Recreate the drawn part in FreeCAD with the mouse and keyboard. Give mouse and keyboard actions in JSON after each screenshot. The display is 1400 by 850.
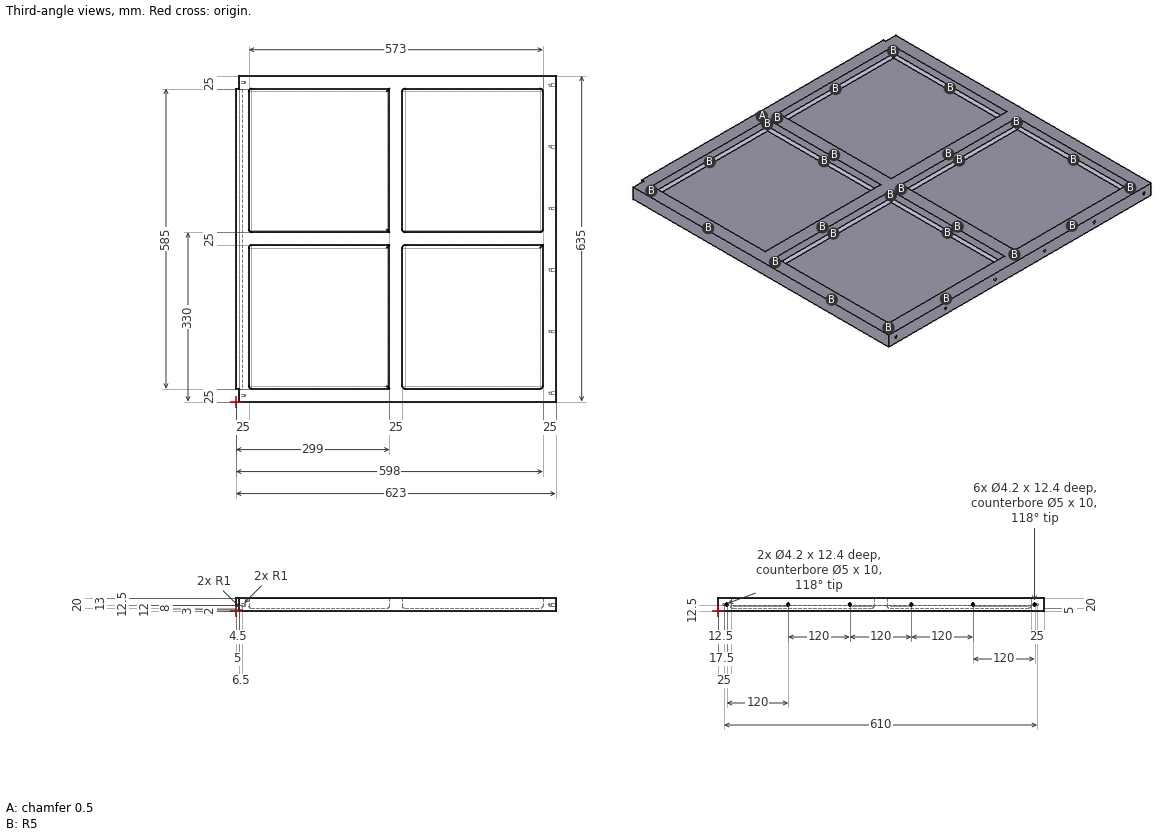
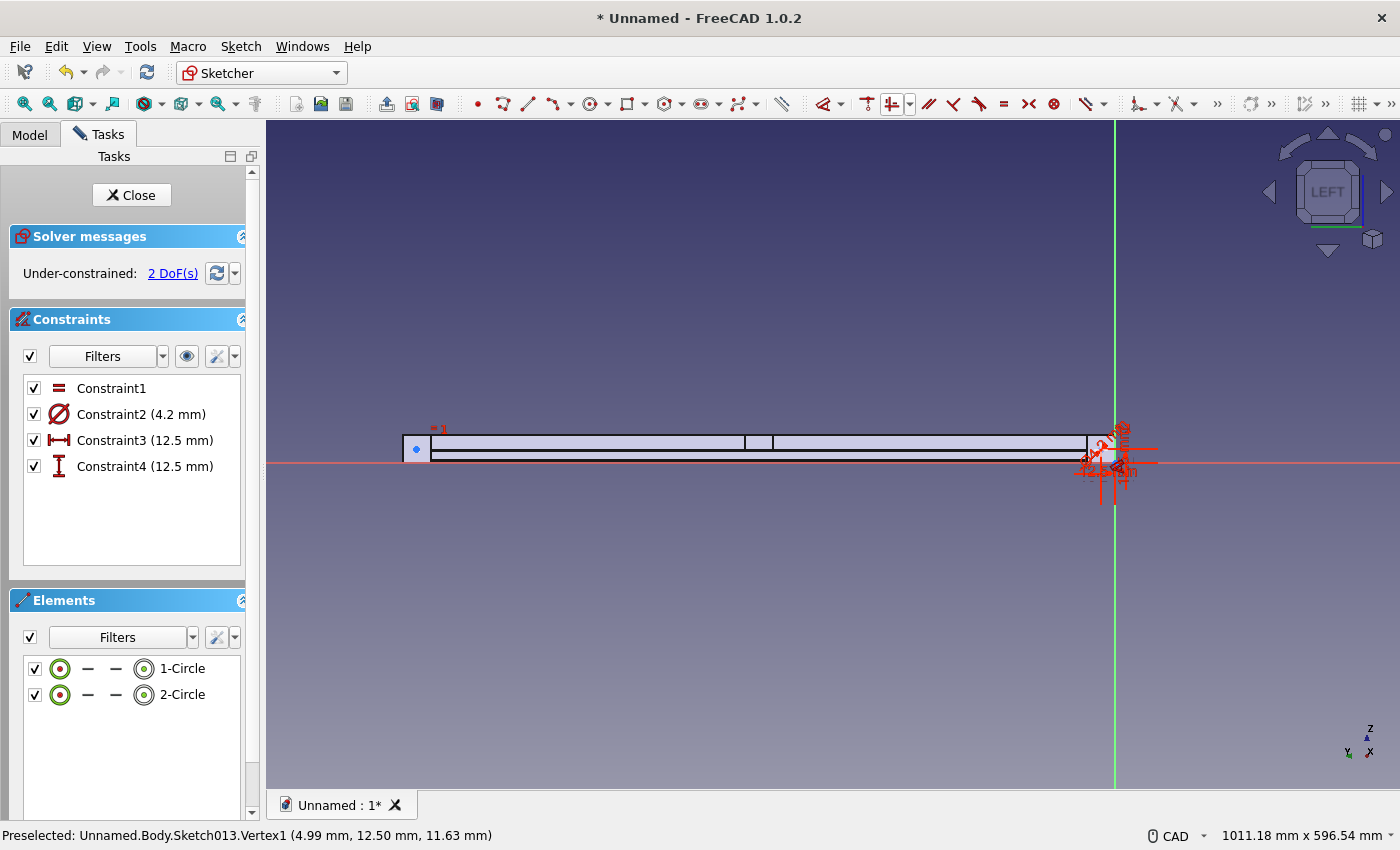
{"action": "scroll", "coordinate": [417, 450], "scroll_direction": "up", "scroll_amount": 6}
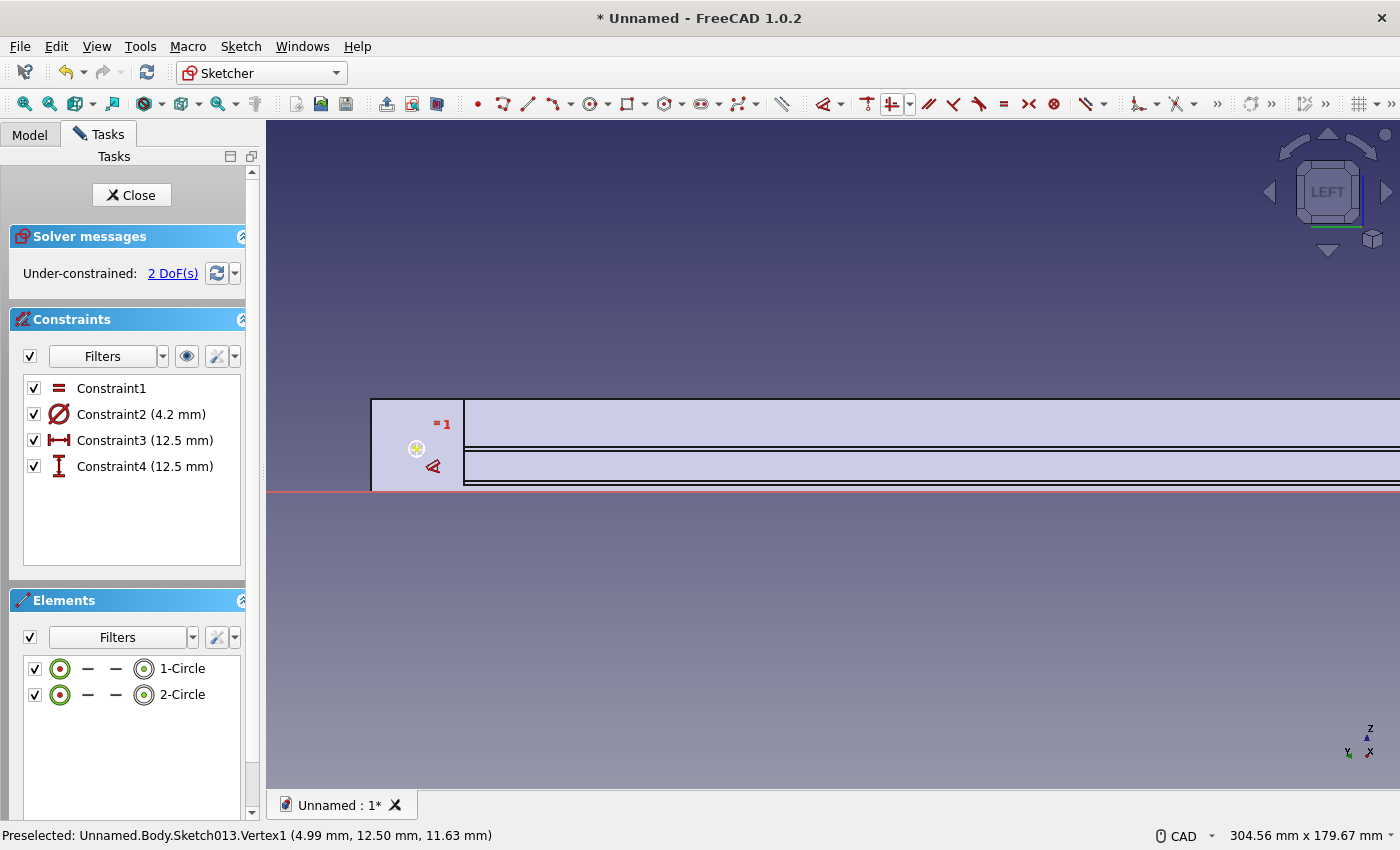
{"action": "left_click", "coordinate": [417, 449]}
{"action": "left_click", "coordinate": [383, 471]}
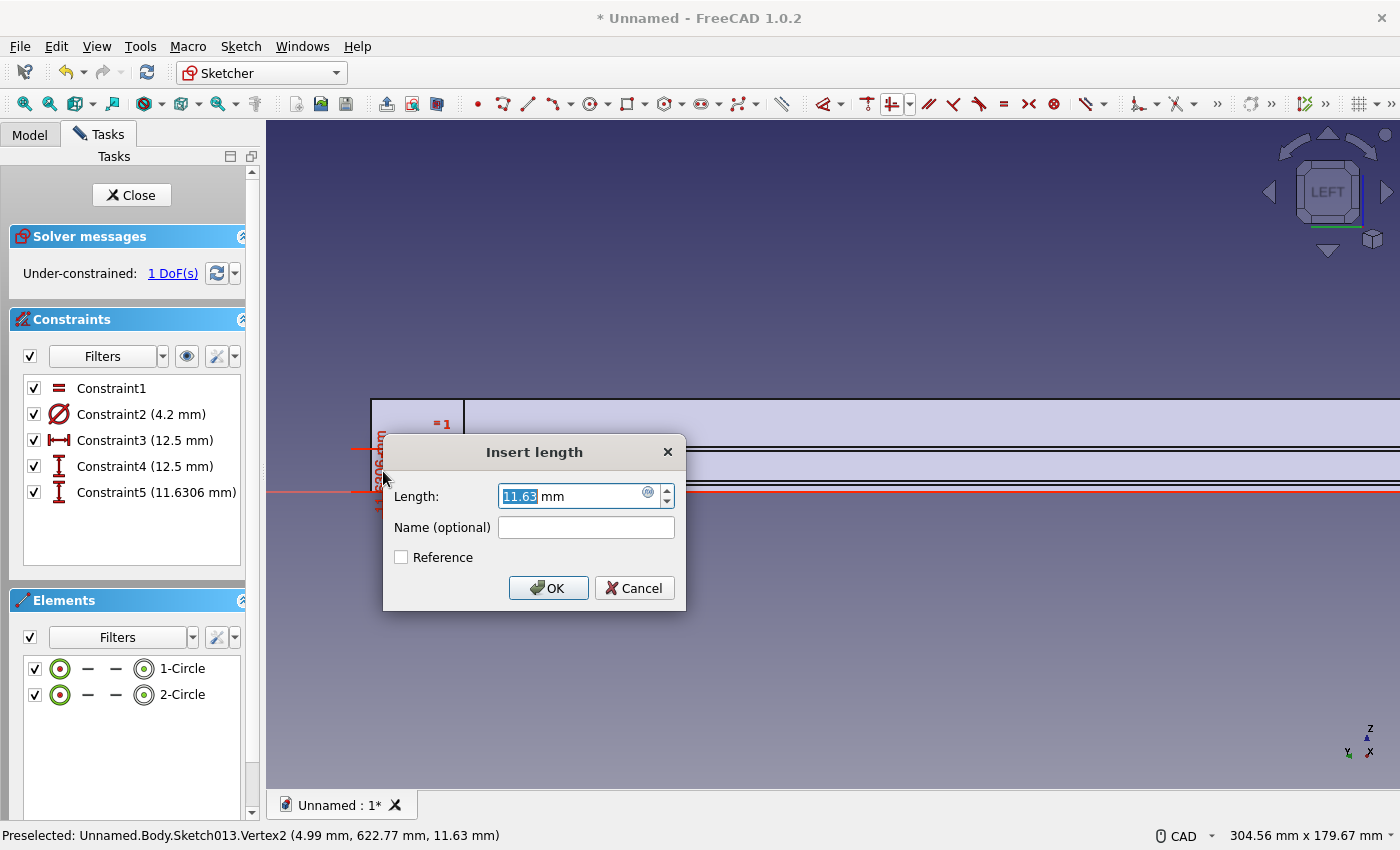
{"action": "type", "text": "12.5"}
{"action": "key", "text": "Return"}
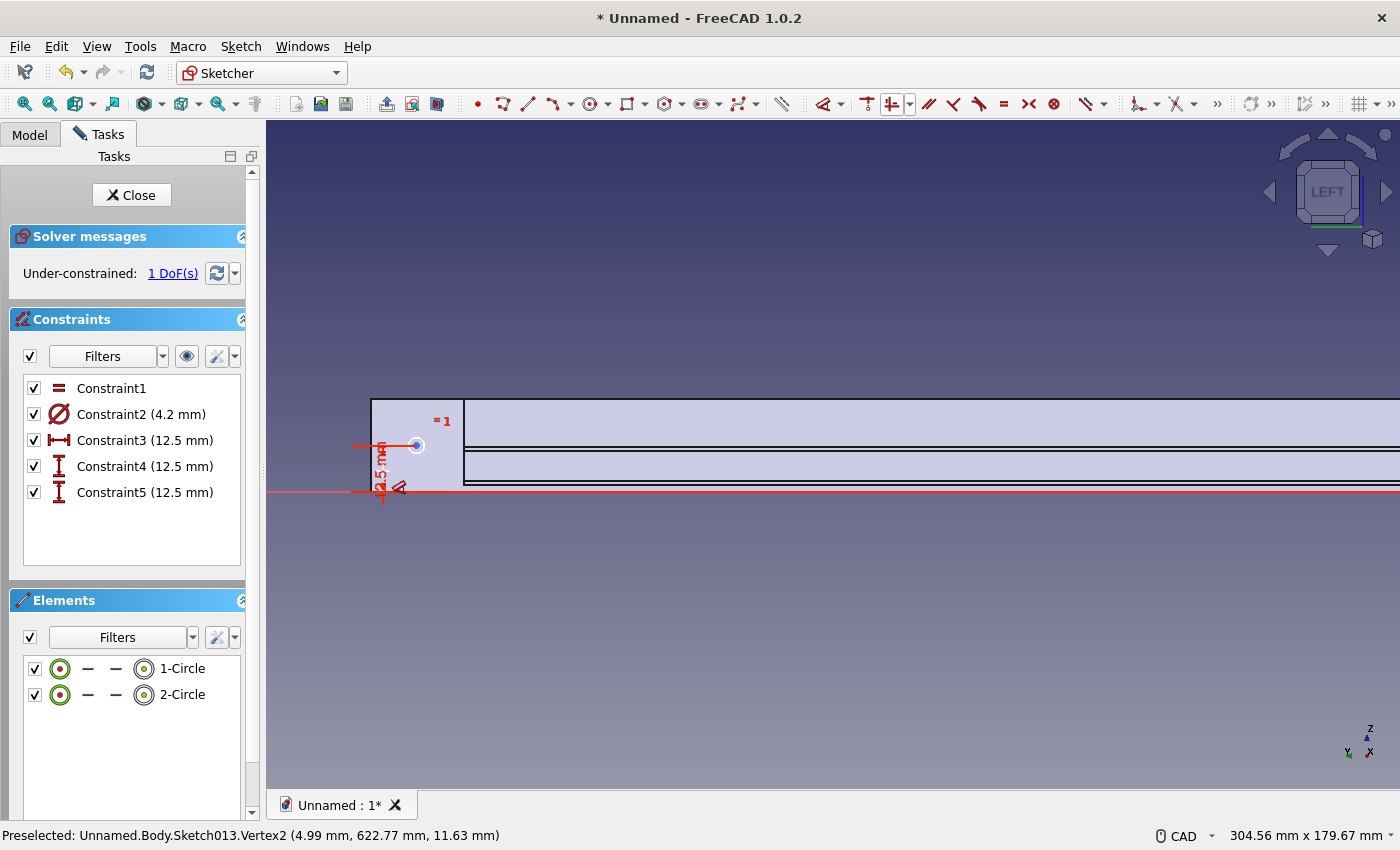
{"action": "scroll", "coordinate": [416, 450], "scroll_direction": "down", "scroll_amount": 6}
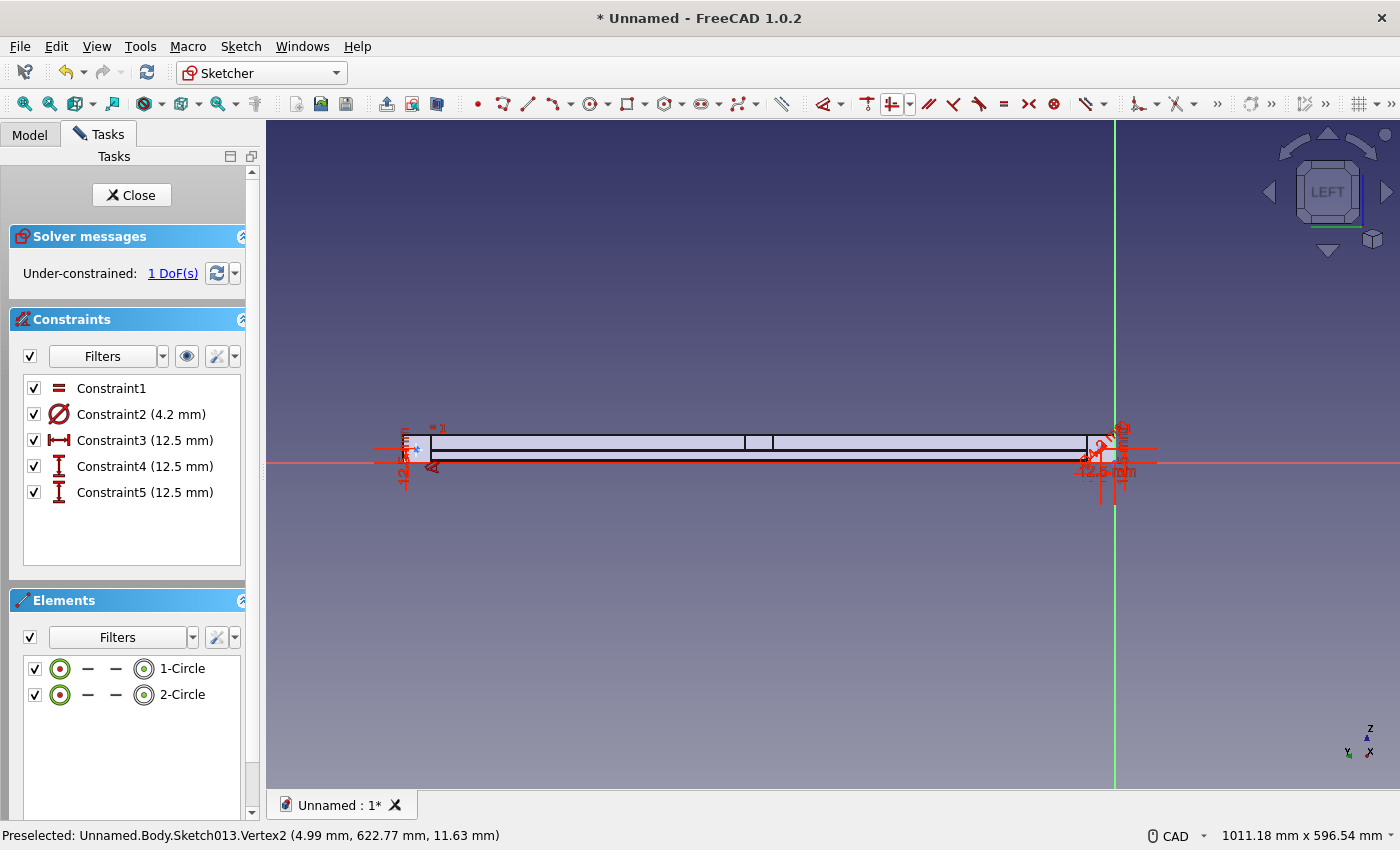
{"action": "left_click", "coordinate": [1101, 449]}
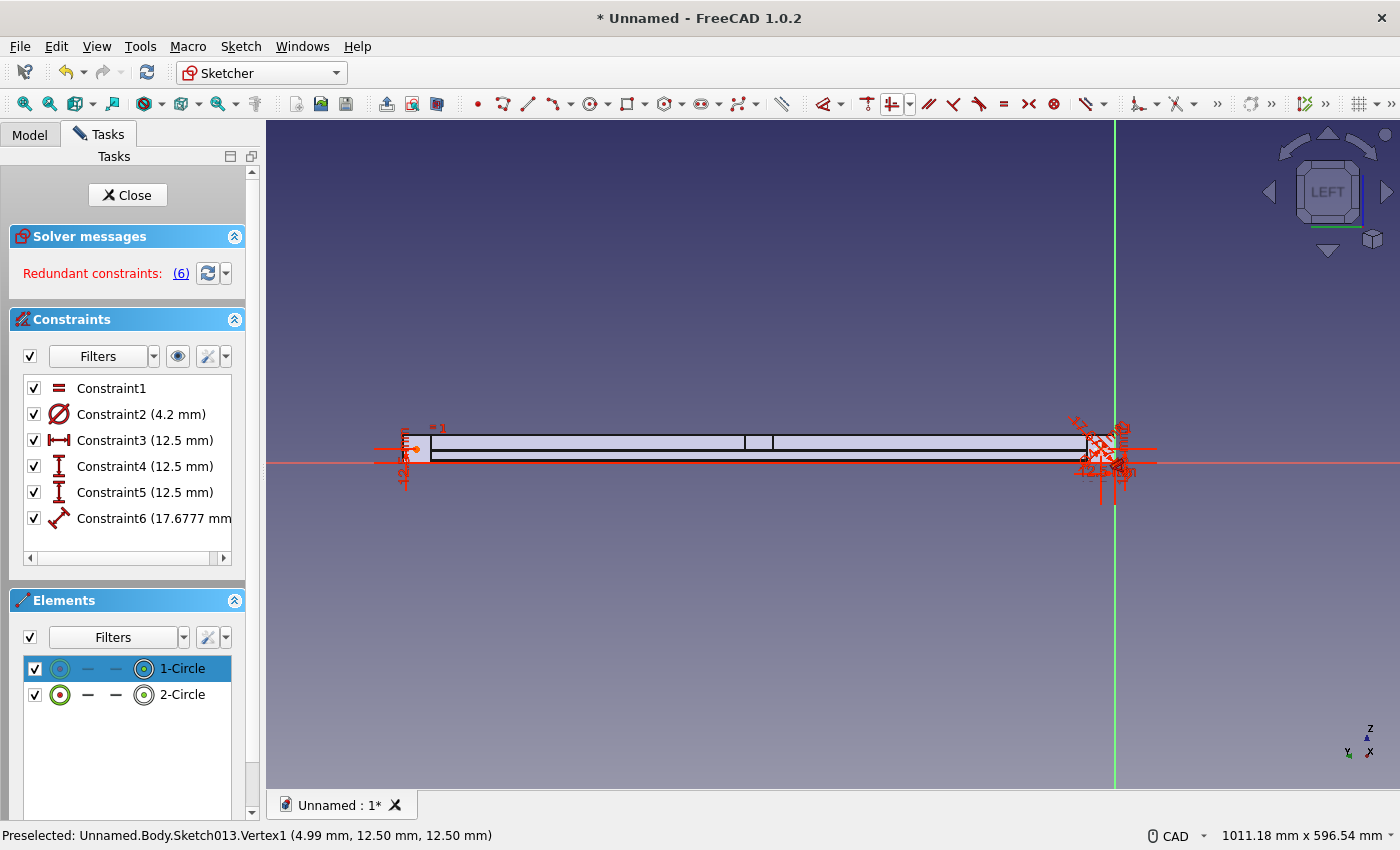
{"action": "left_click", "coordinate": [416, 449]}
{"action": "left_click", "coordinate": [758, 415]}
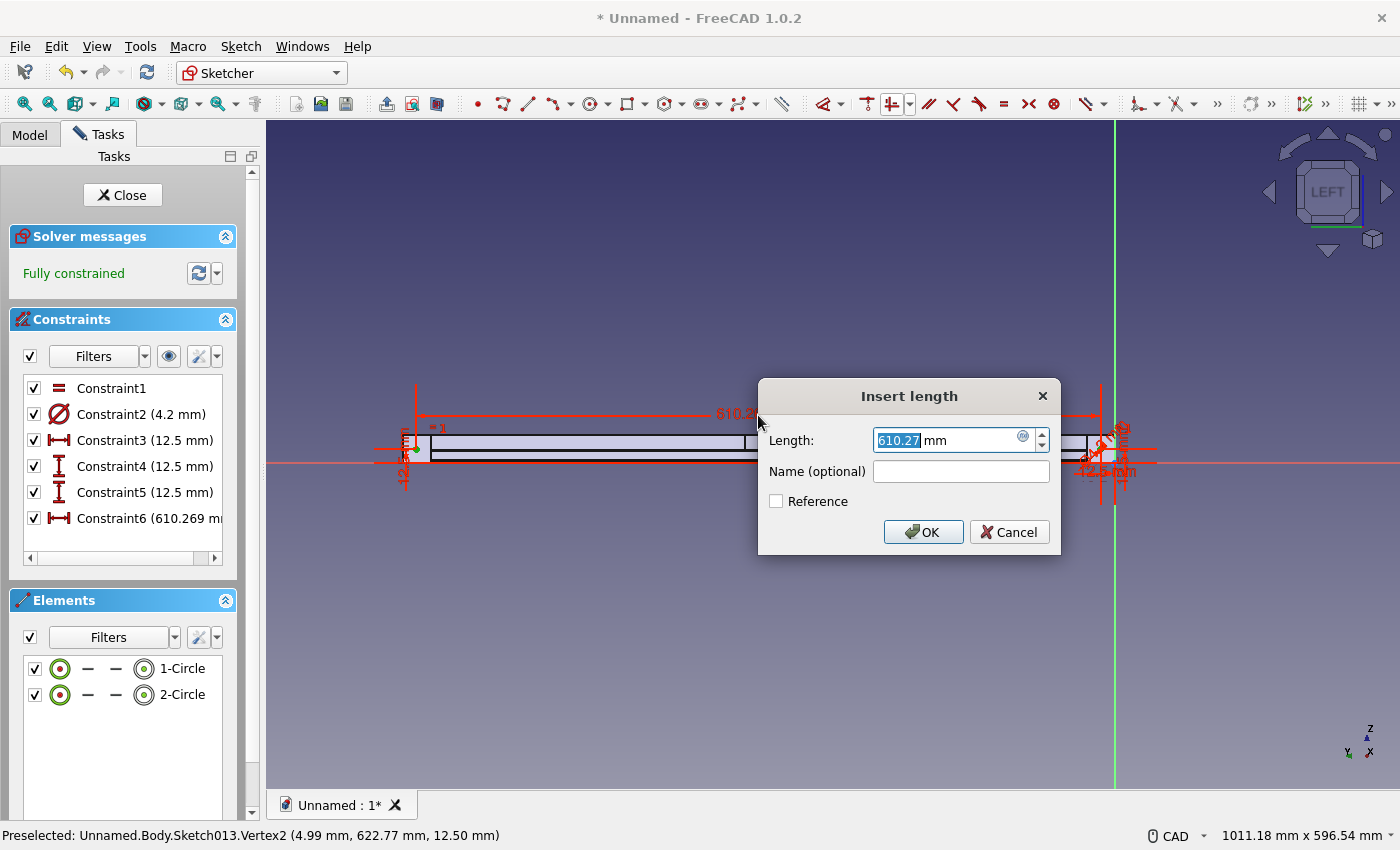
{"action": "type", "text": "610"}
{"action": "key", "text": "Return"}
{"action": "key", "text": "Escape"}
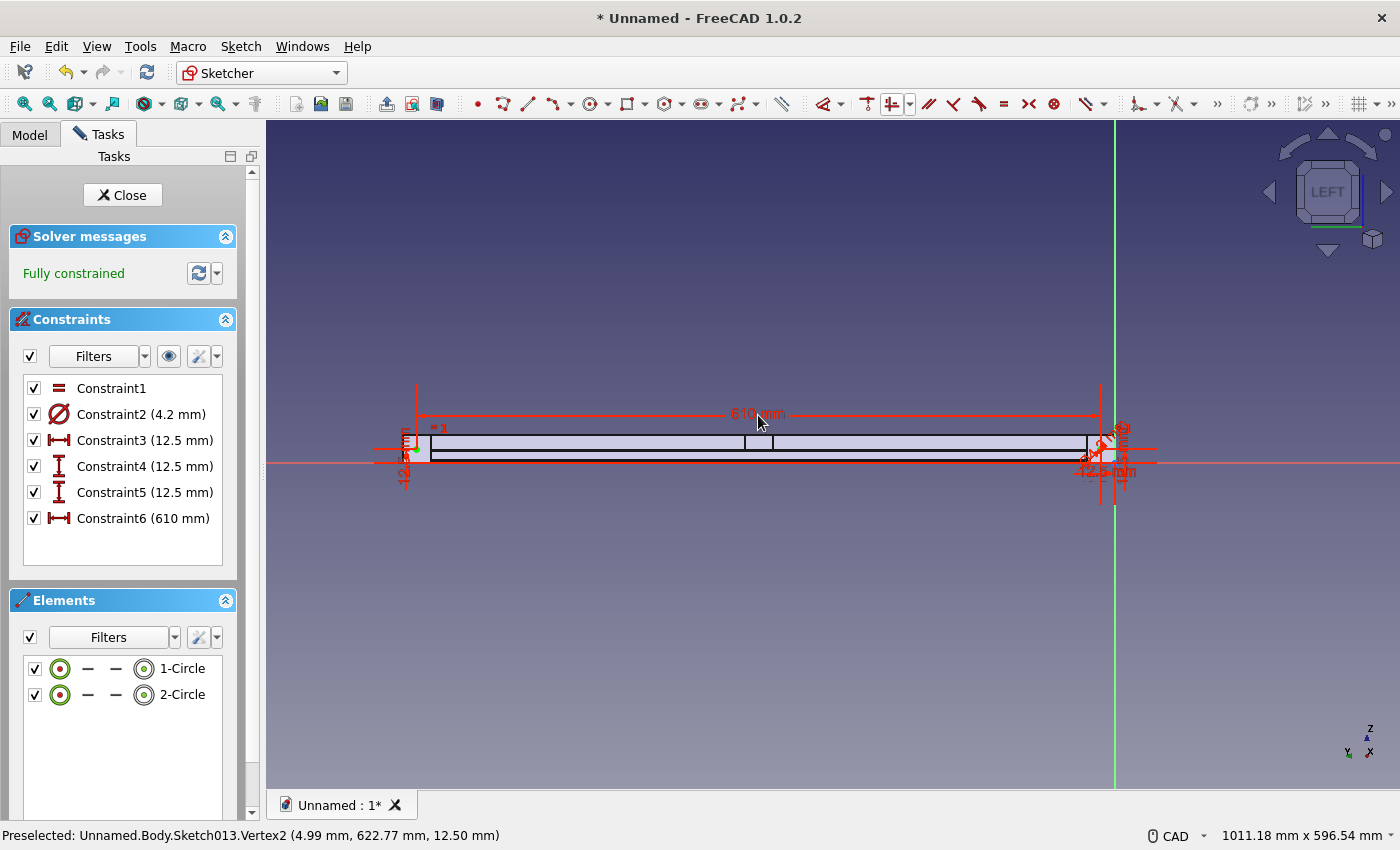
{"action": "left_click", "coordinate": [123, 195]}